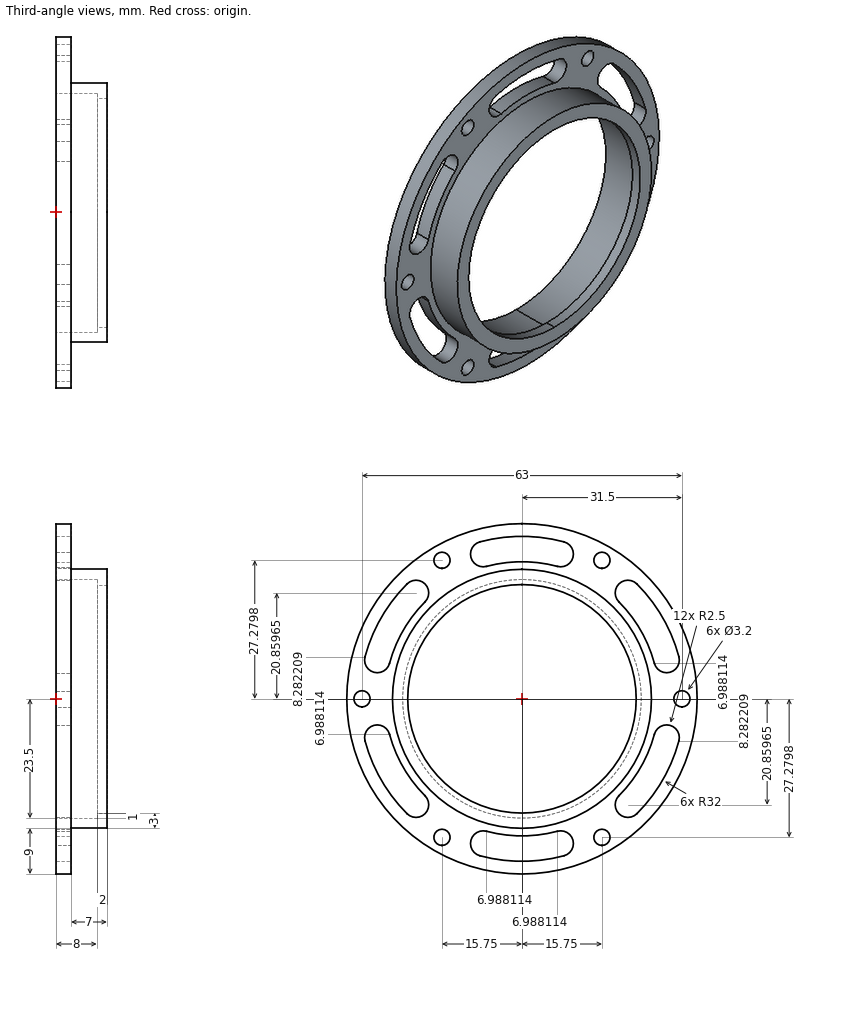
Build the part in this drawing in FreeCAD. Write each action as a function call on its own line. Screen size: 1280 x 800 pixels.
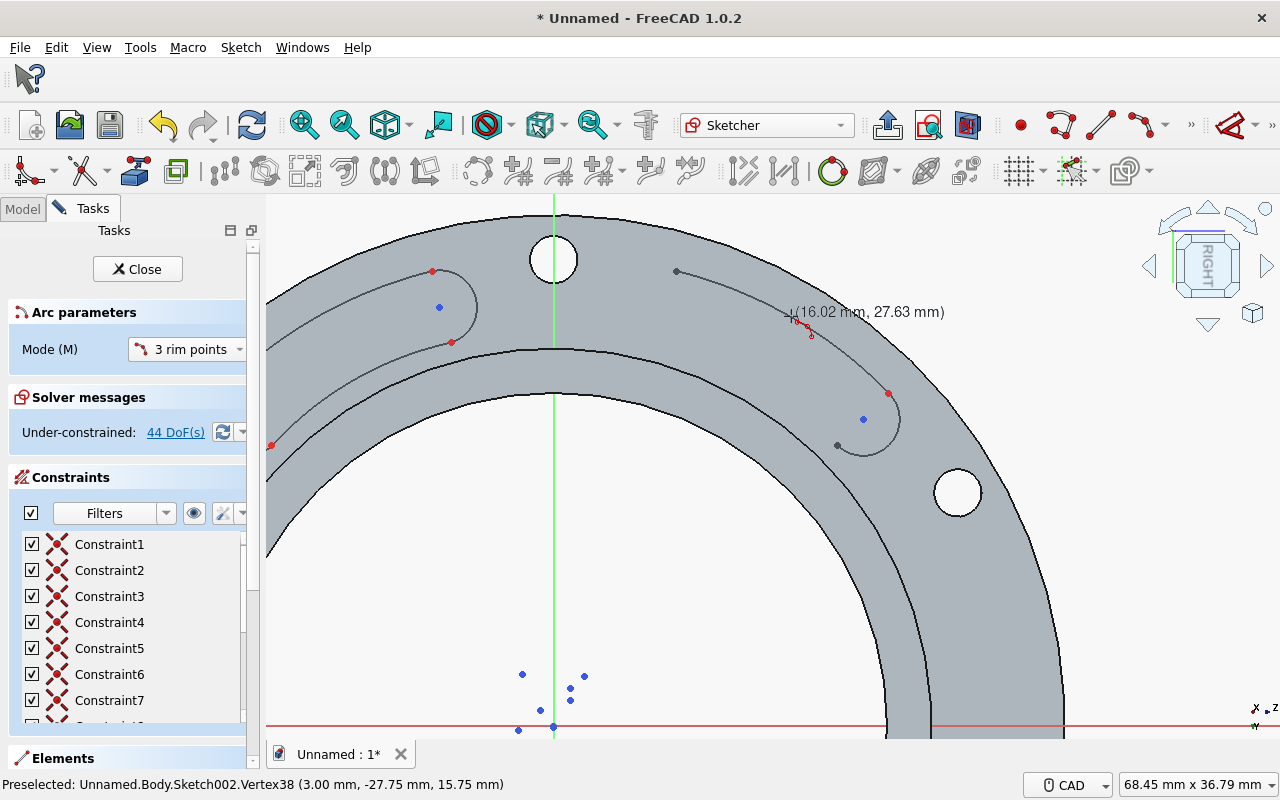
click(677, 271)
click(657, 340)
click(631, 295)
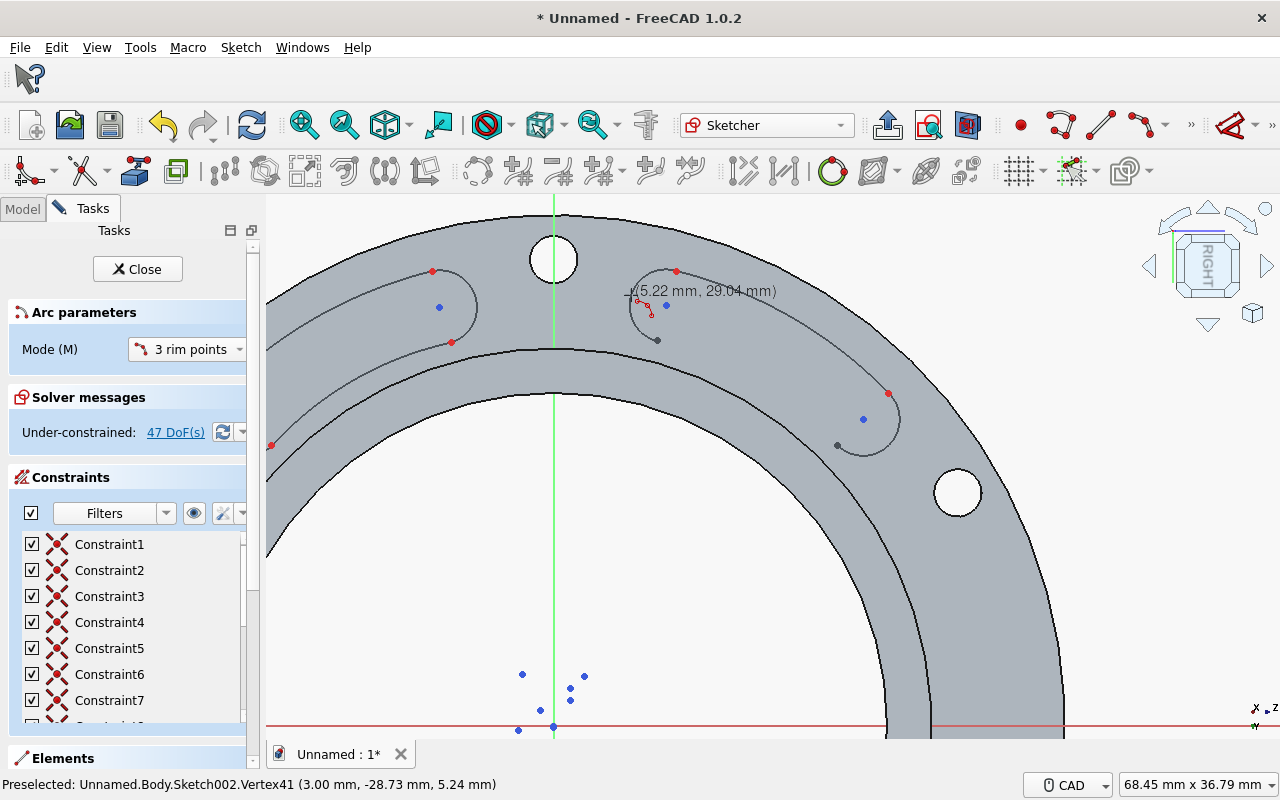
click(657, 341)
click(837, 445)
click(754, 380)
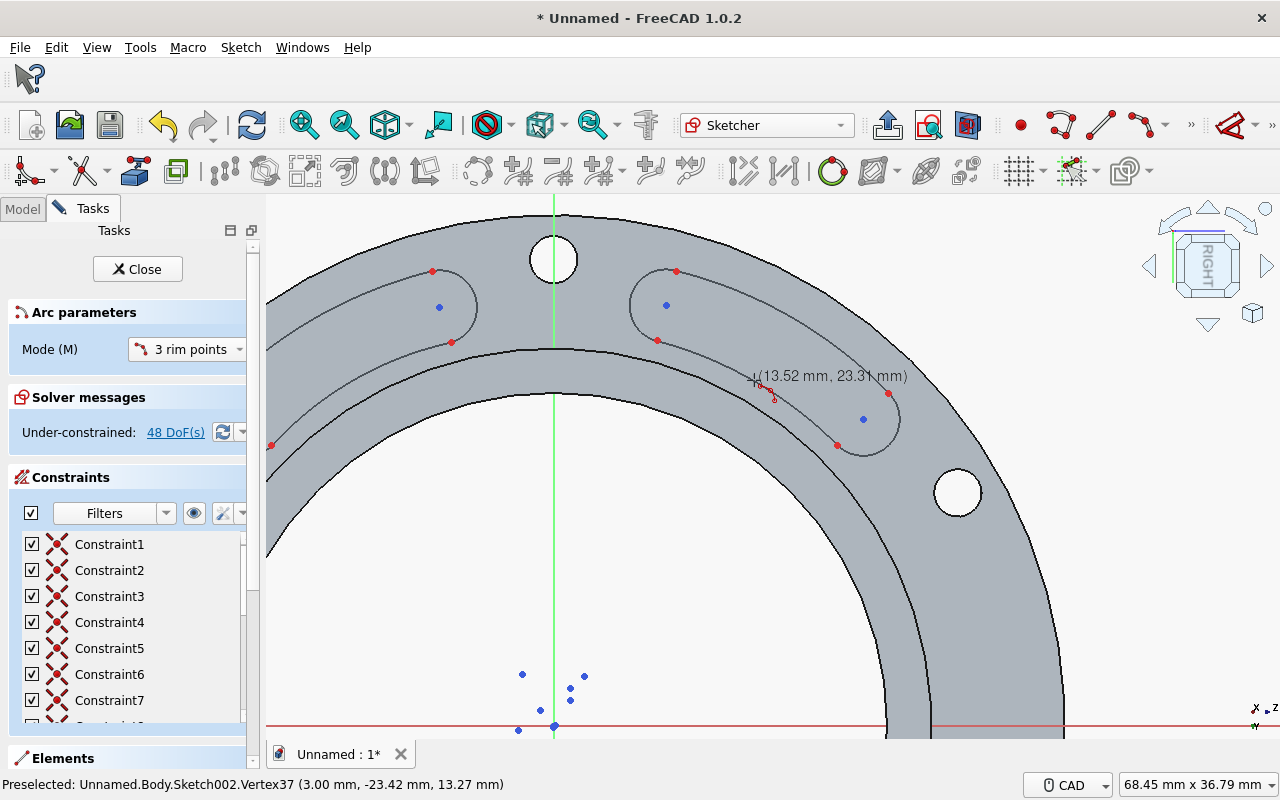
click(940, 623)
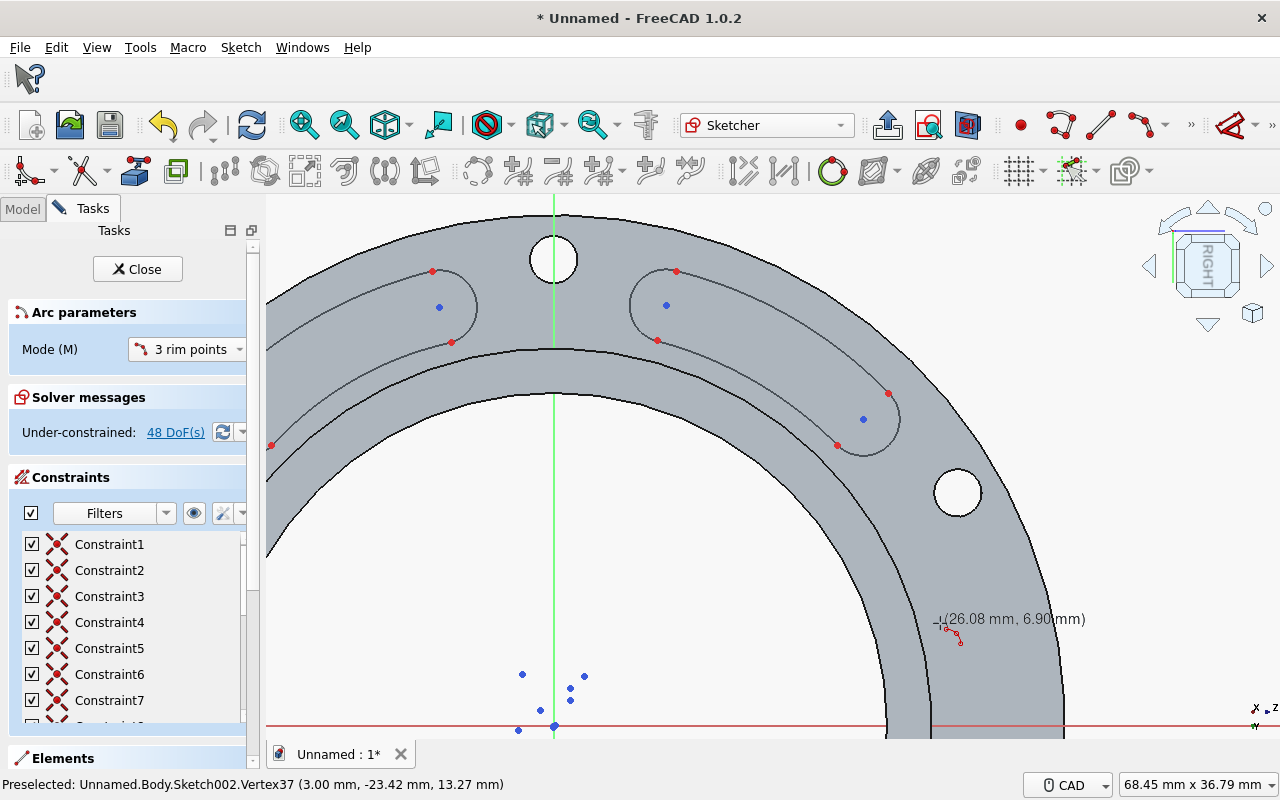
scroll(792, 315, down, 5)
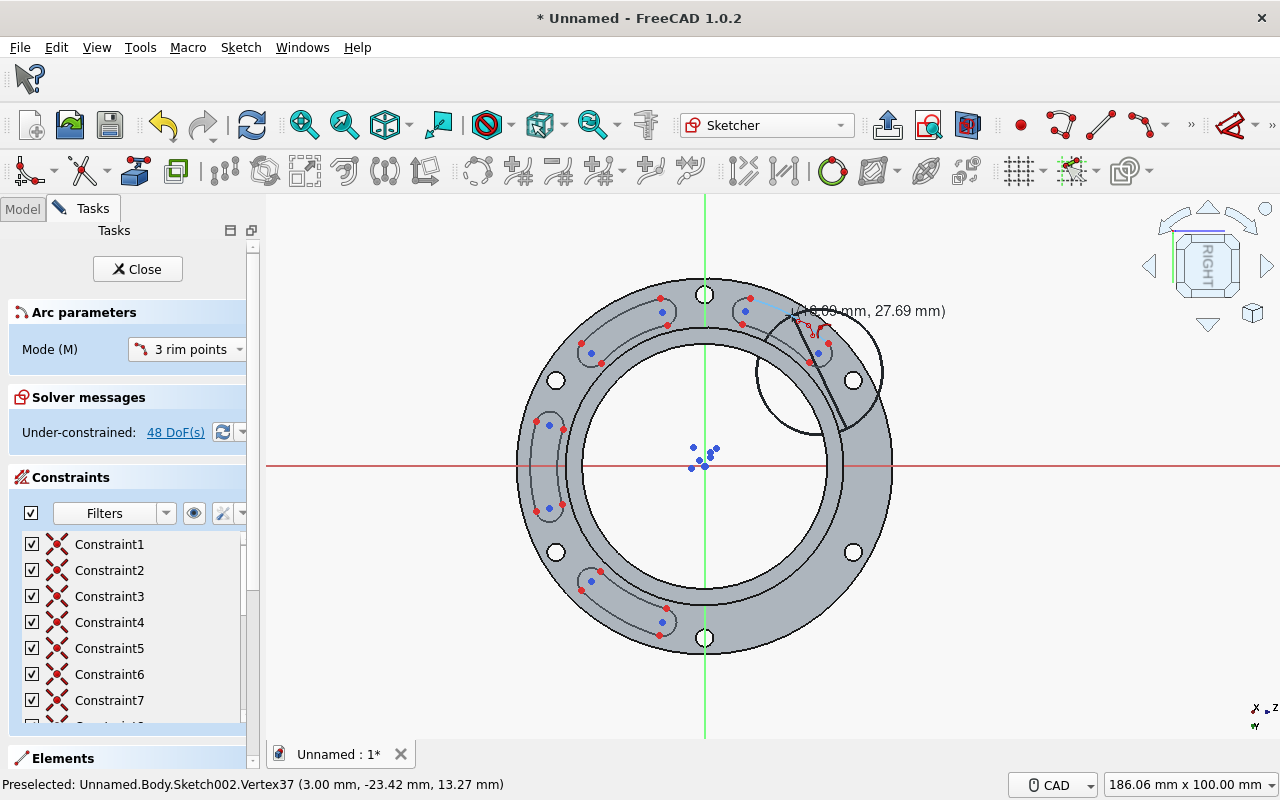
click(847, 505)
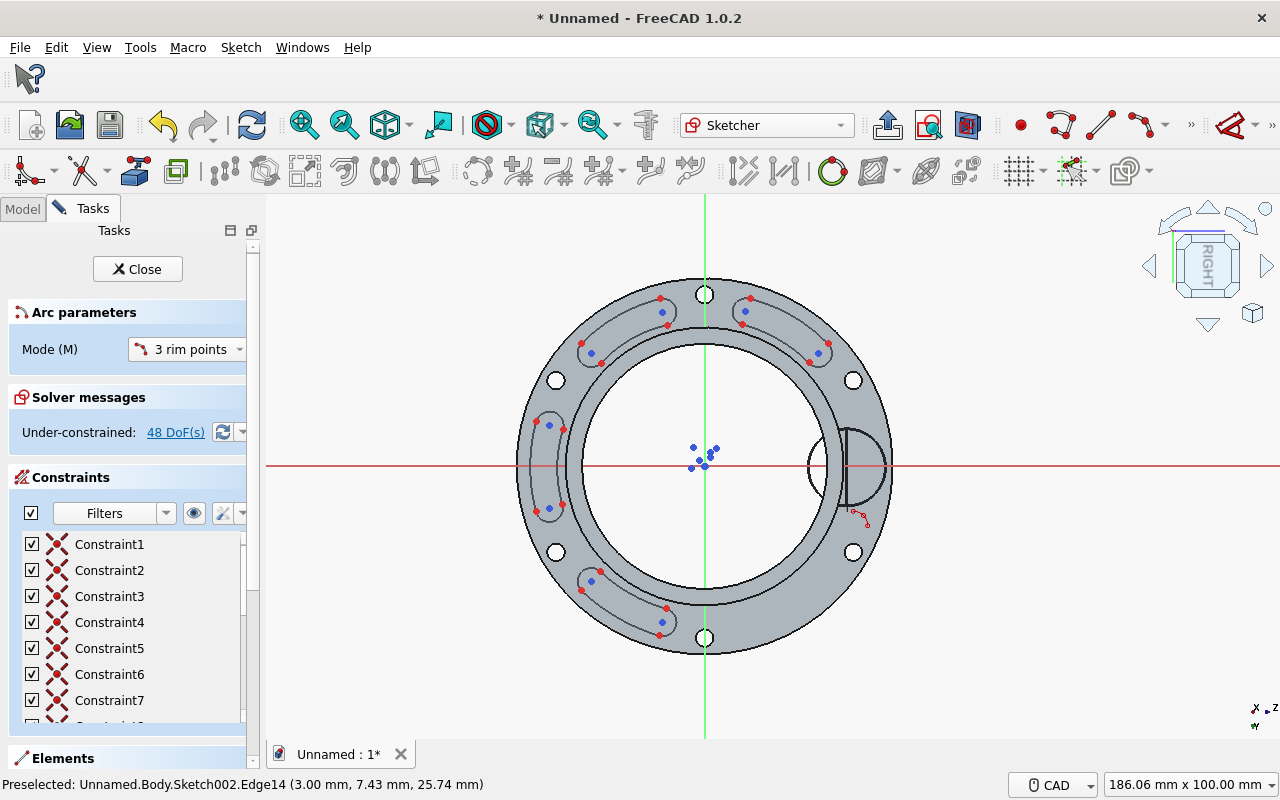
scroll(852, 474, up, 6)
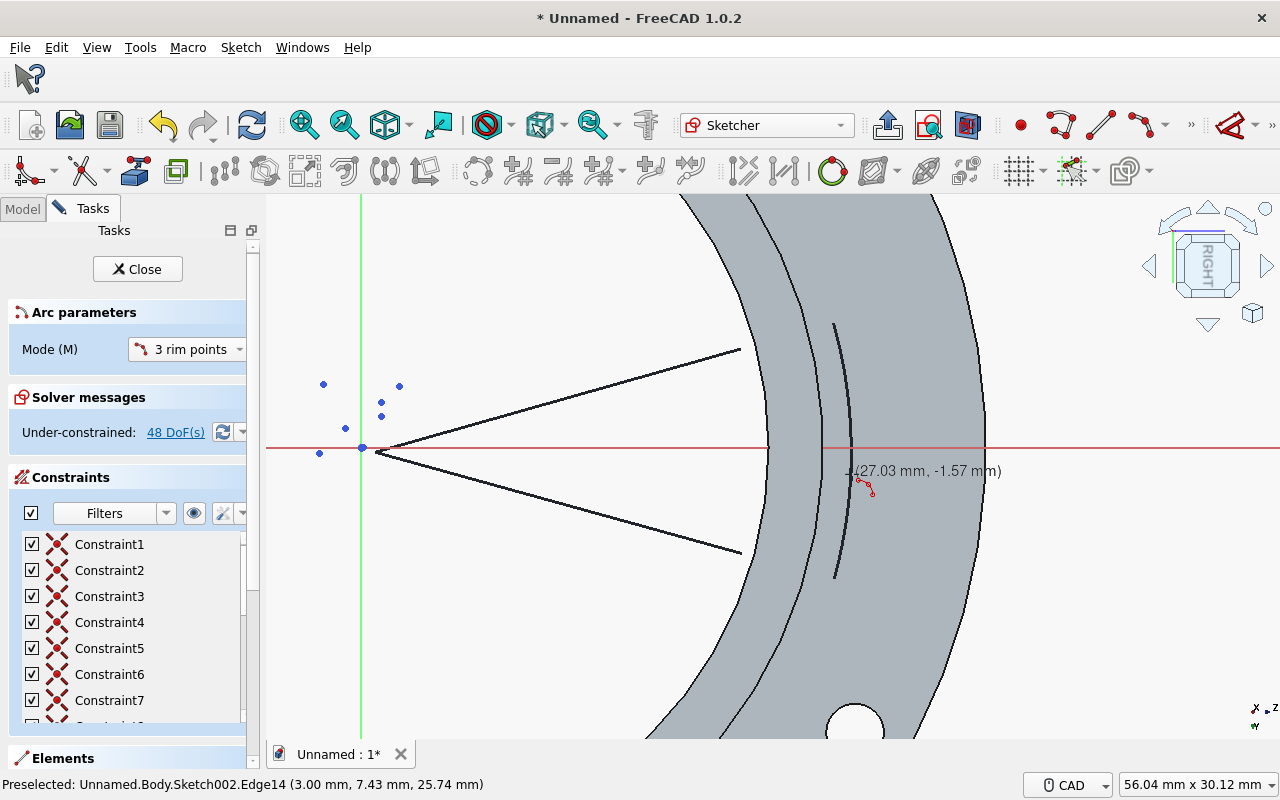
click(849, 473)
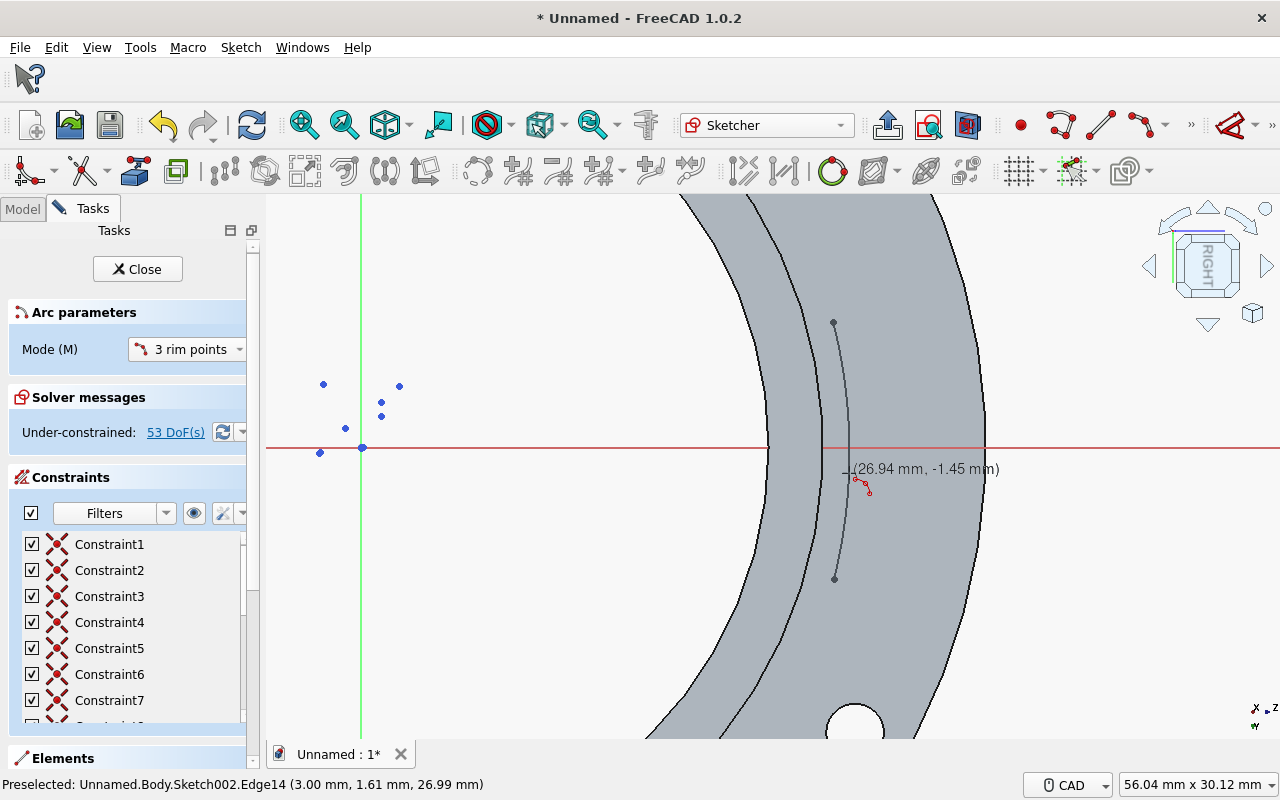
click(834, 579)
click(921, 598)
click(865, 630)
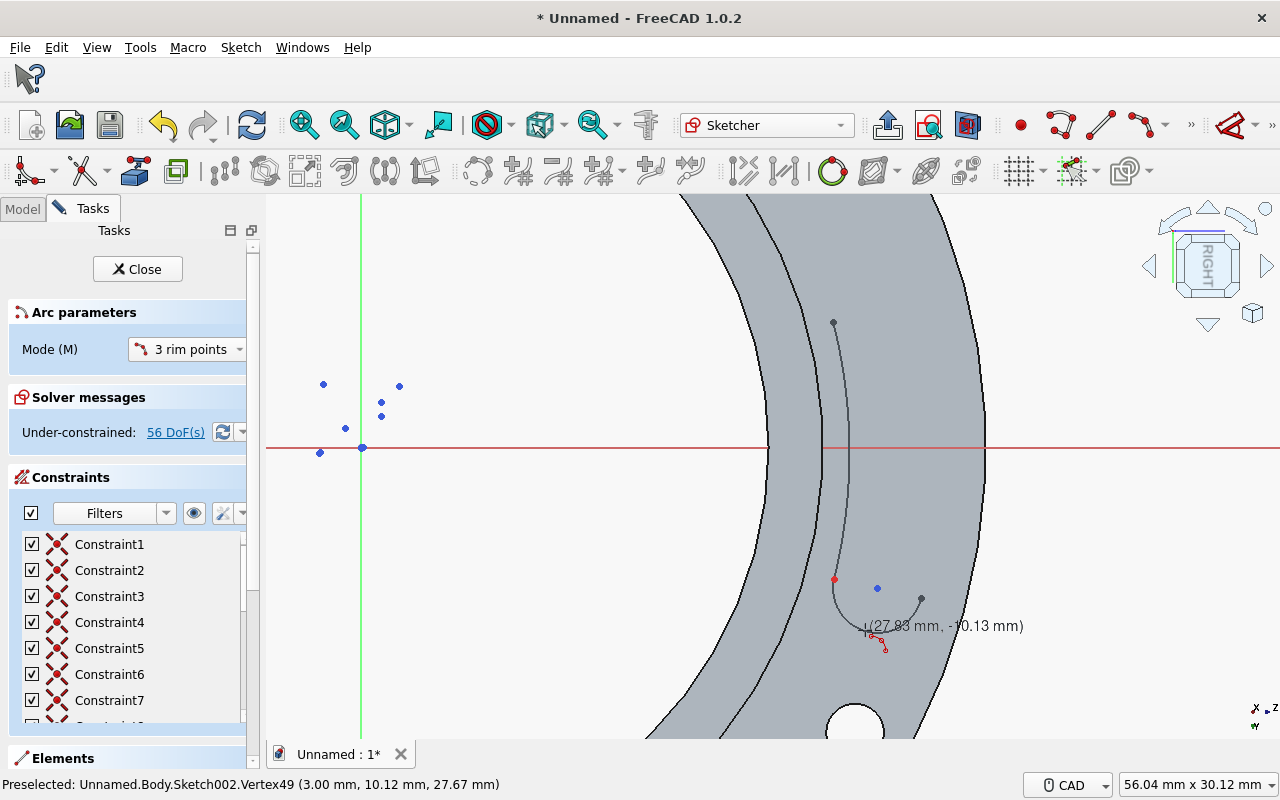
click(921, 599)
click(921, 298)
click(940, 478)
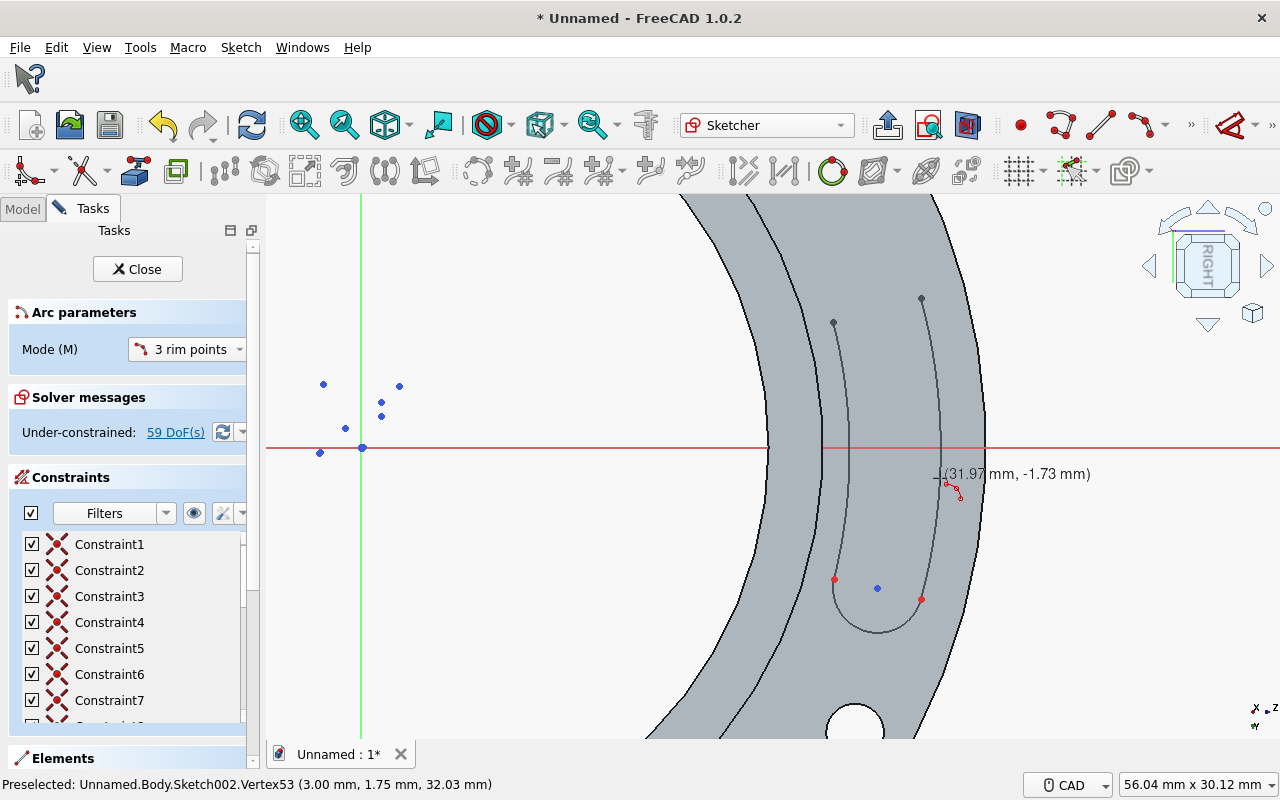
click(921, 299)
click(833, 323)
click(865, 266)